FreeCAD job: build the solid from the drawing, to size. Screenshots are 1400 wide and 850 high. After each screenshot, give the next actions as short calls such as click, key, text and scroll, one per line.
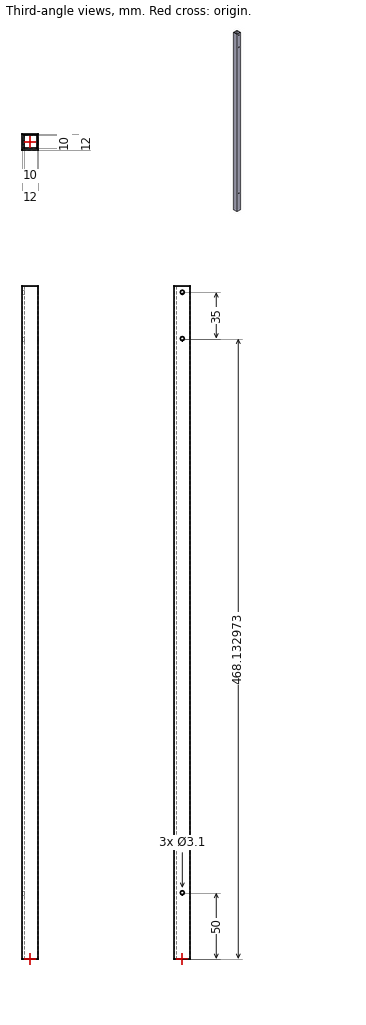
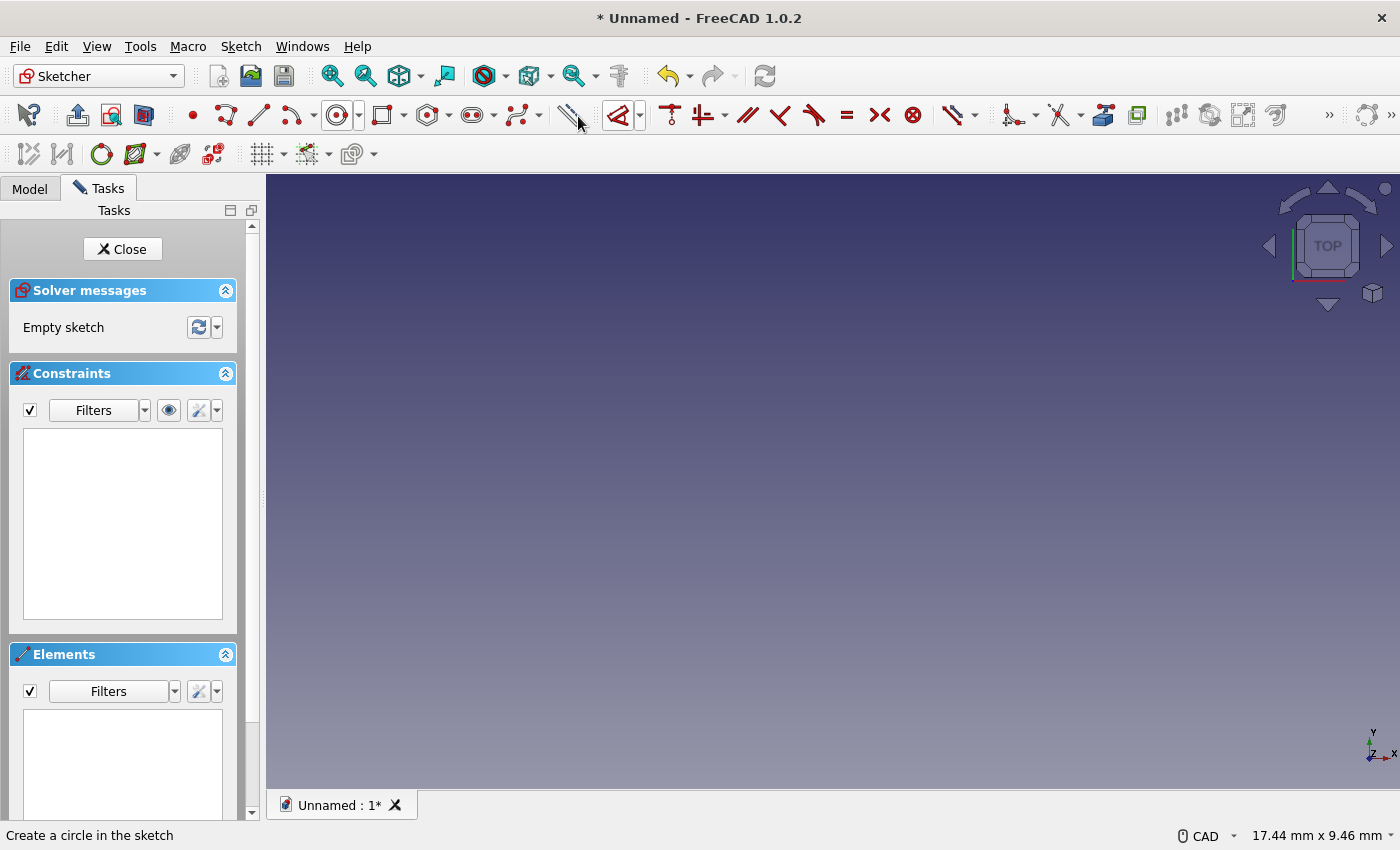
scroll(764, 482, down, 5)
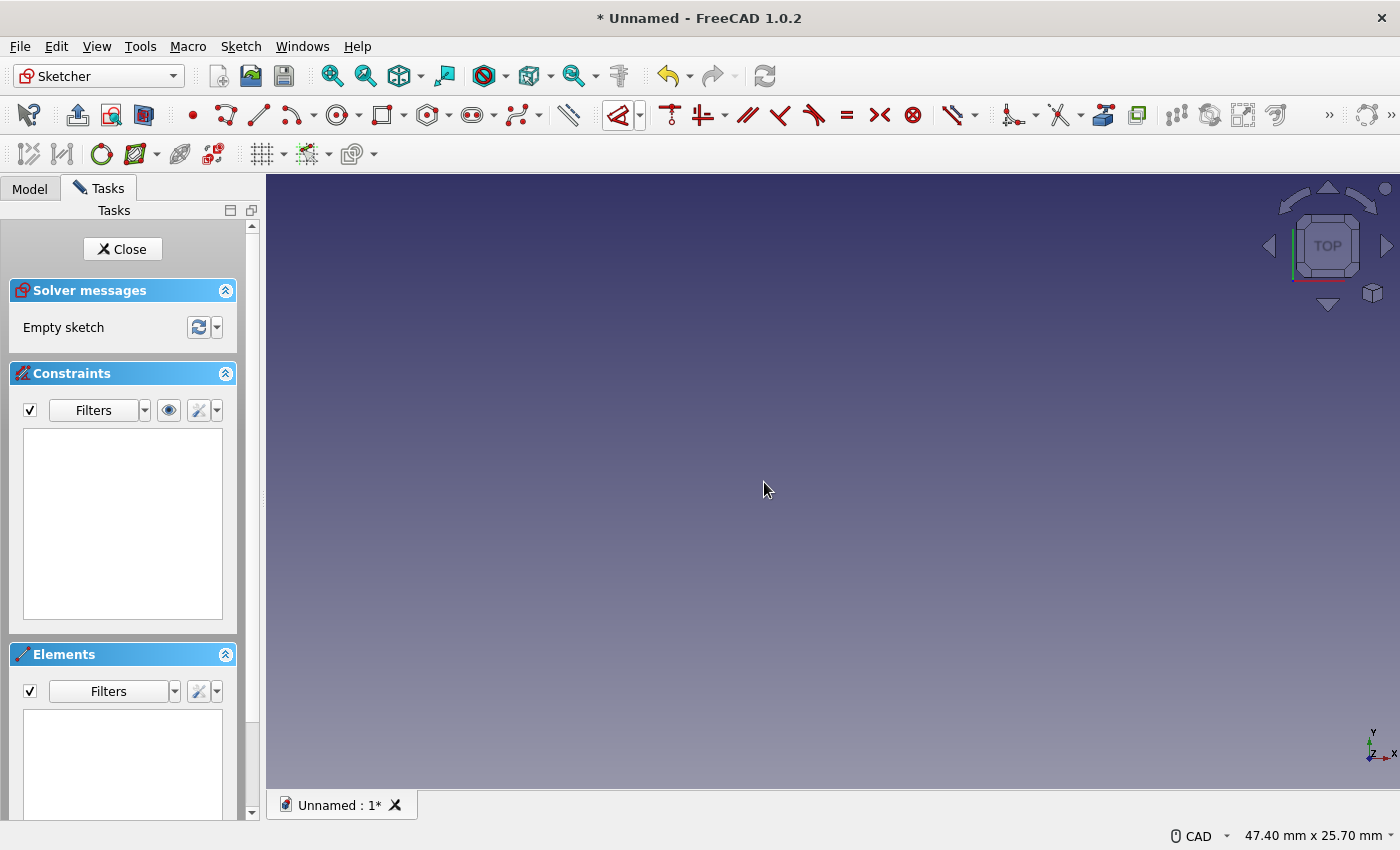
scroll(764, 482, down, 5)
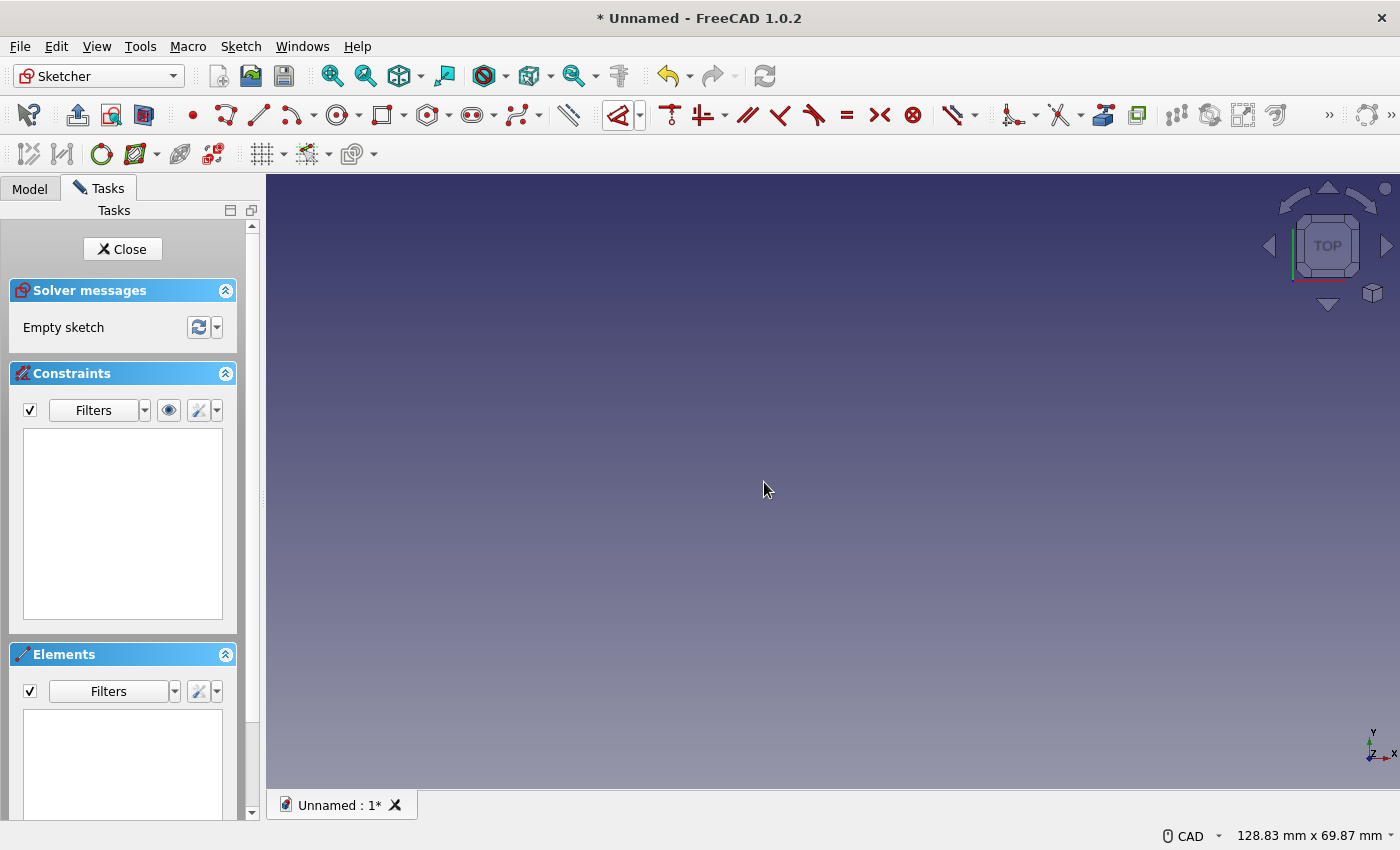
scroll(764, 482, down, 5)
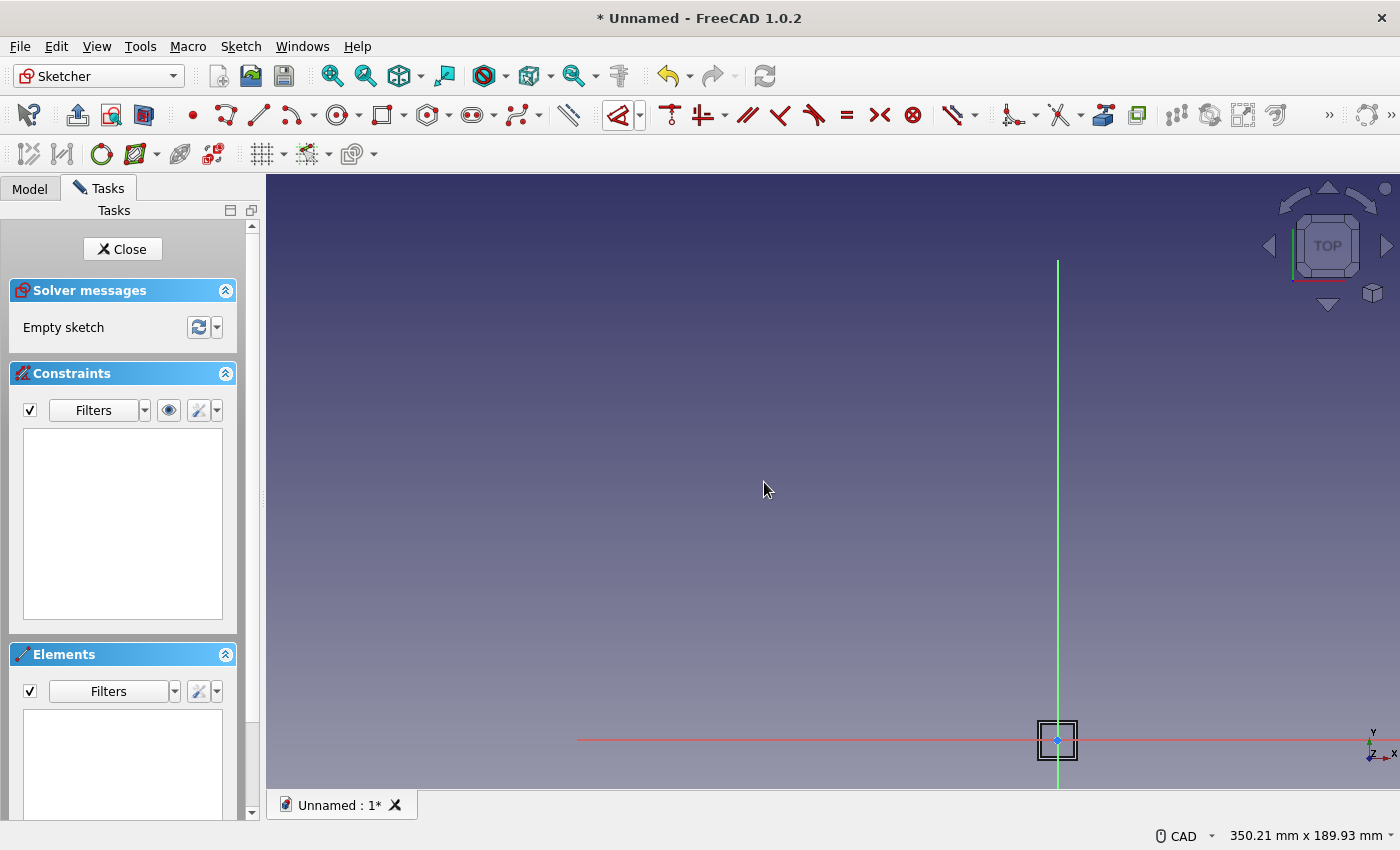
scroll(764, 482, down, 5)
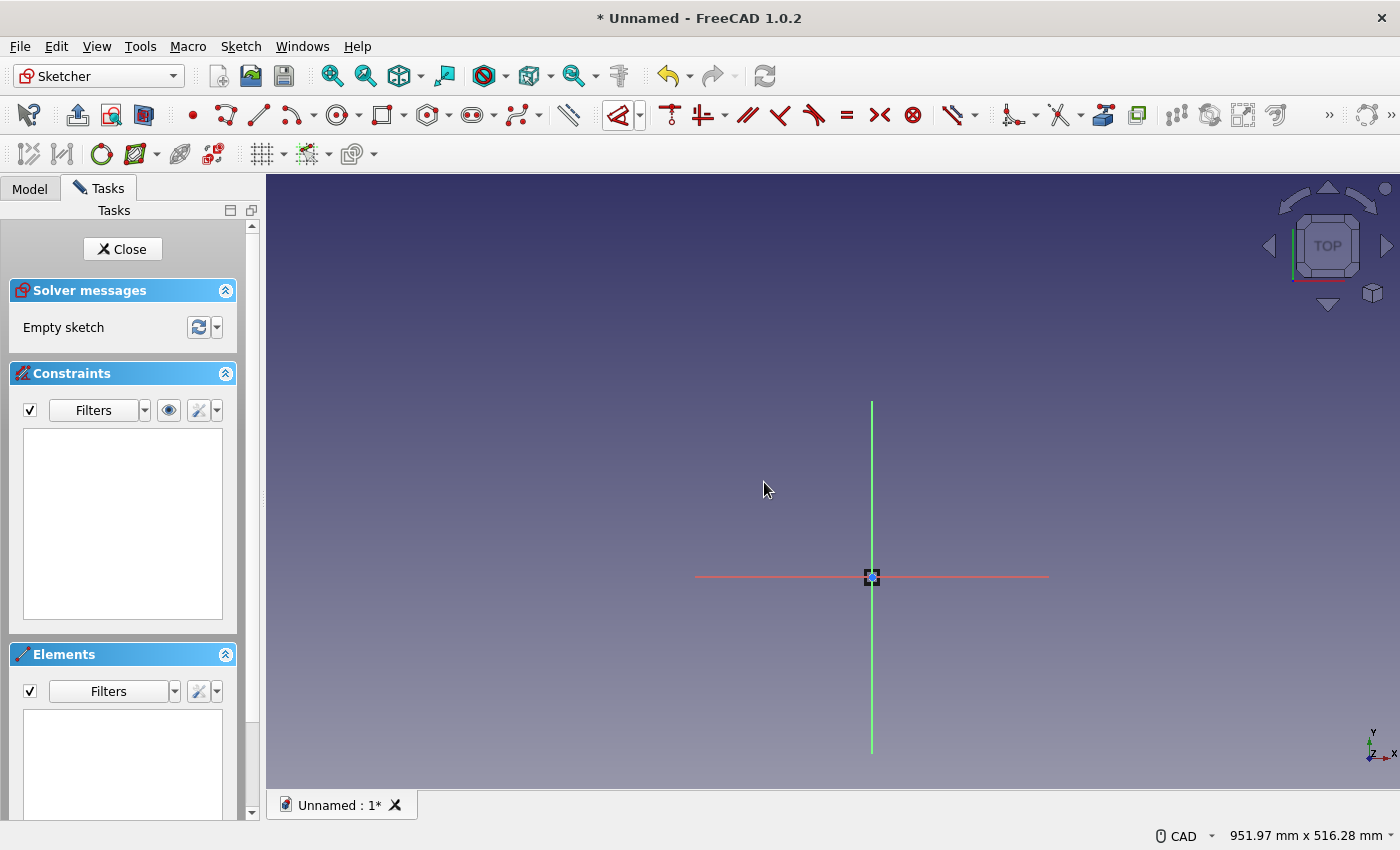
scroll(878, 582, up, 15)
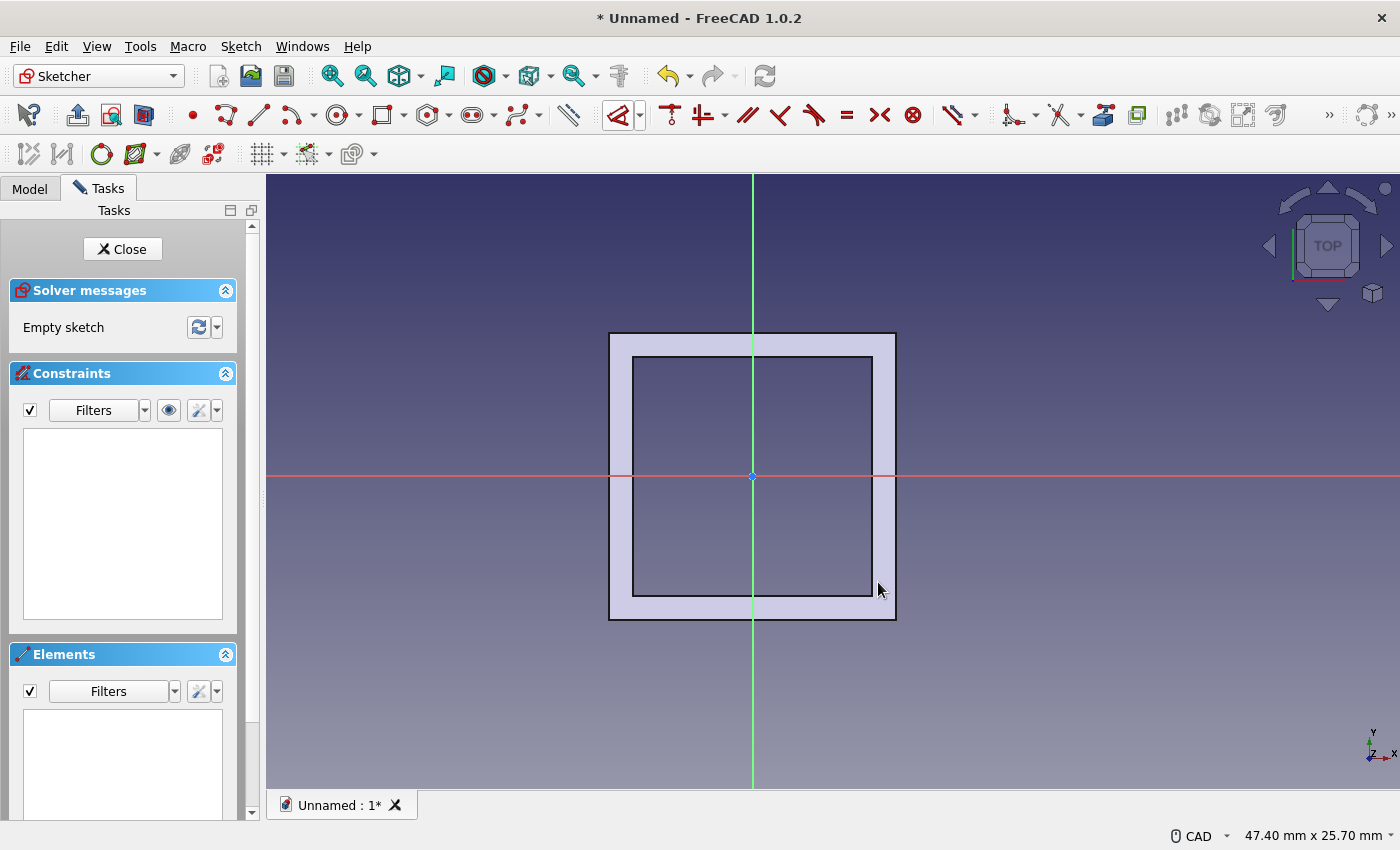
click(404, 116)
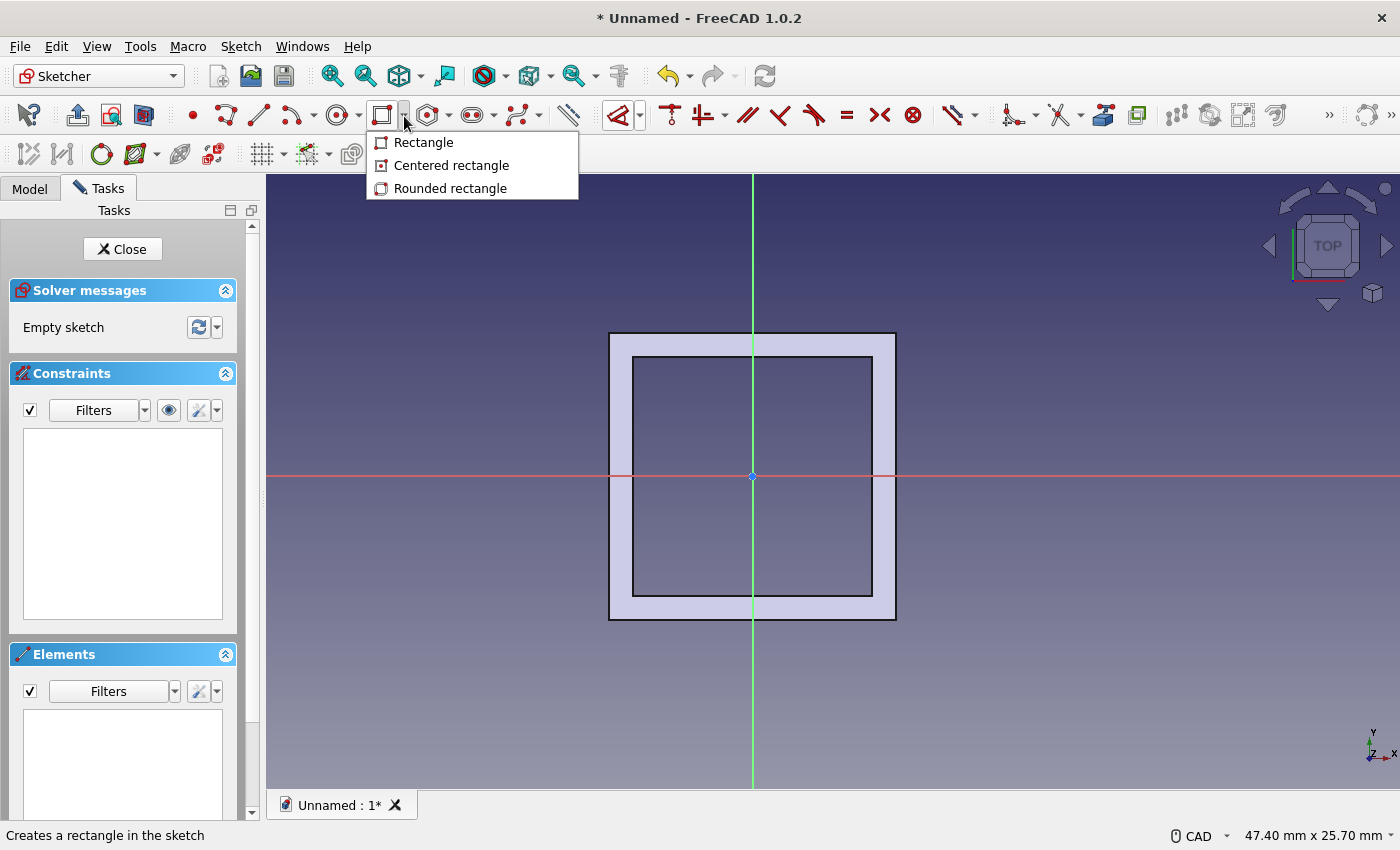
click(472, 166)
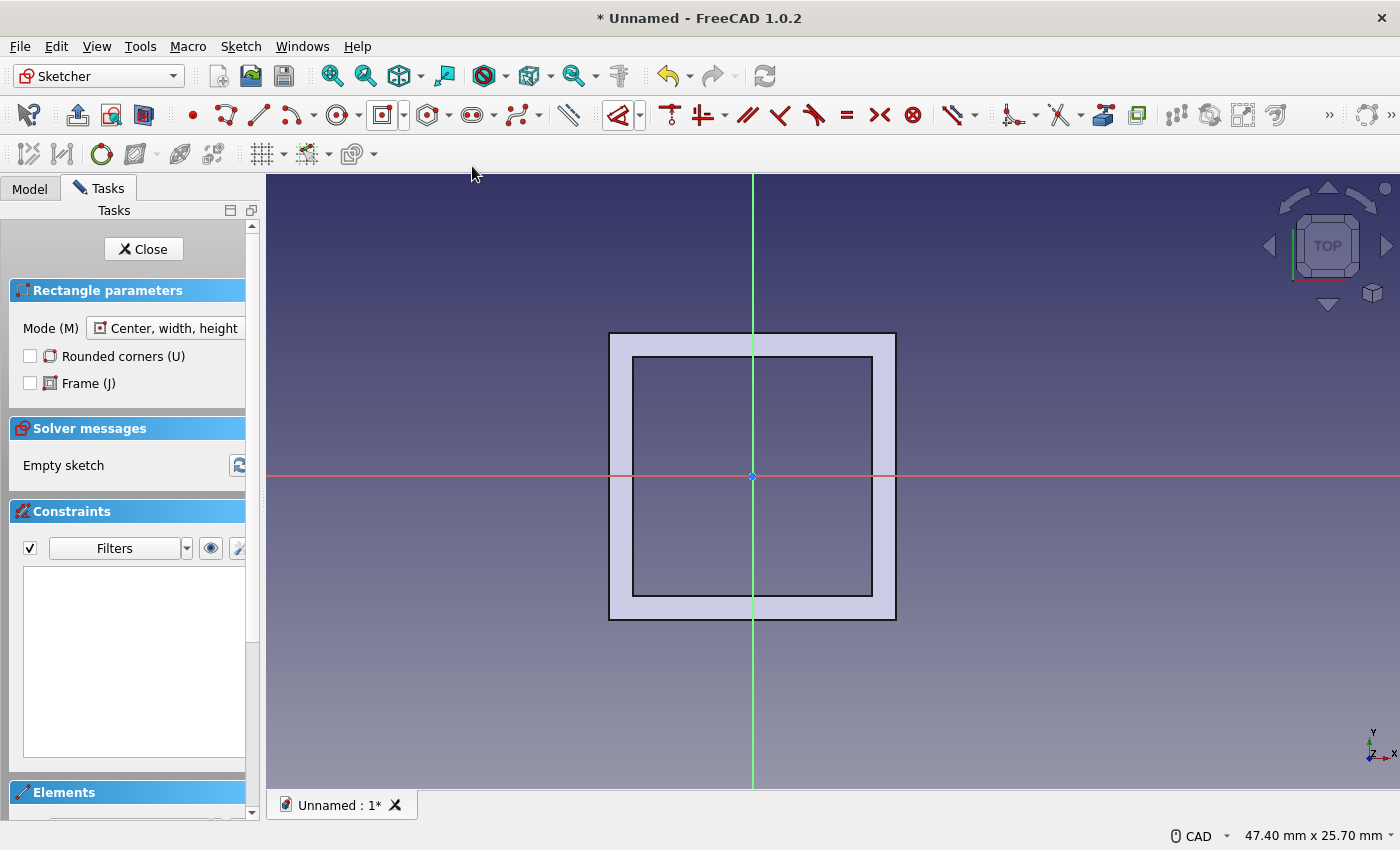
click(753, 476)
click(896, 333)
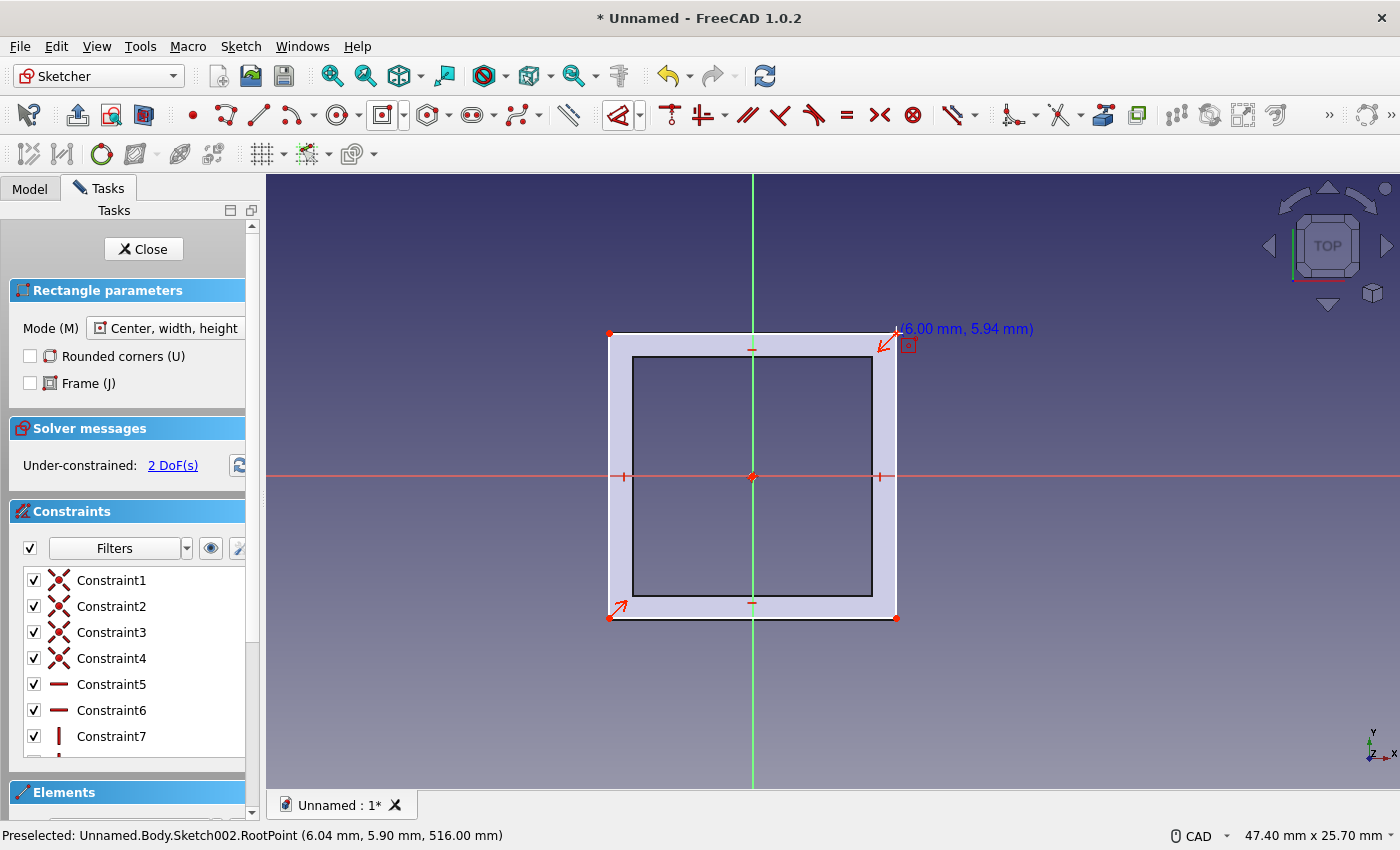
click(753, 476)
click(872, 357)
key(Escape)